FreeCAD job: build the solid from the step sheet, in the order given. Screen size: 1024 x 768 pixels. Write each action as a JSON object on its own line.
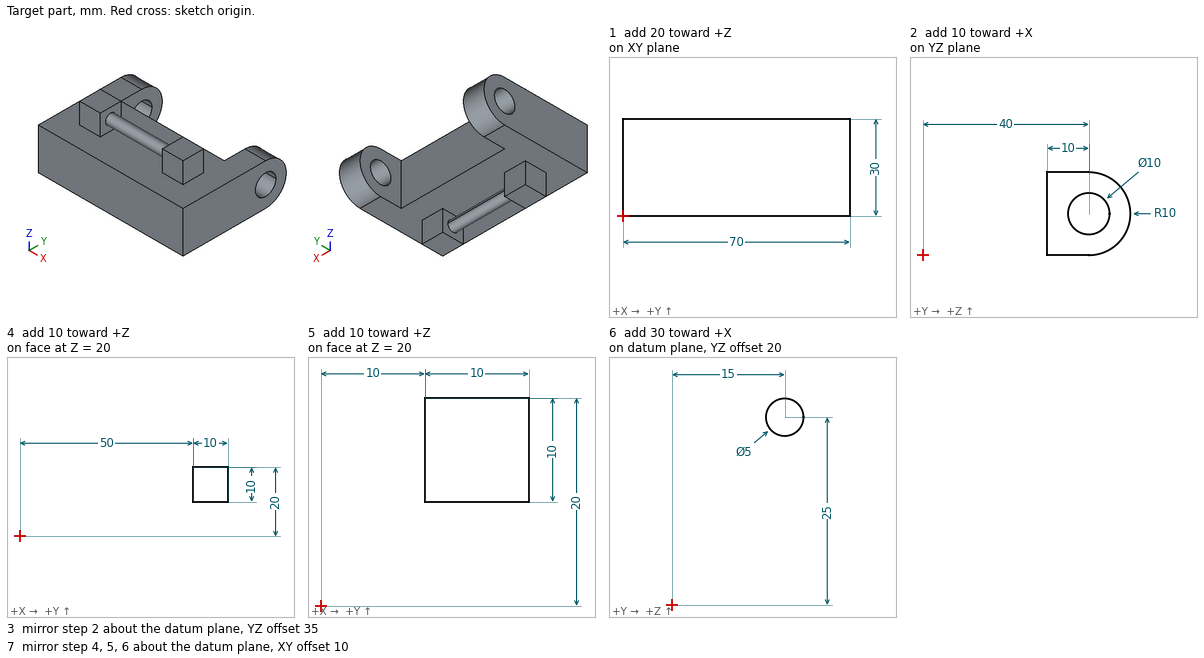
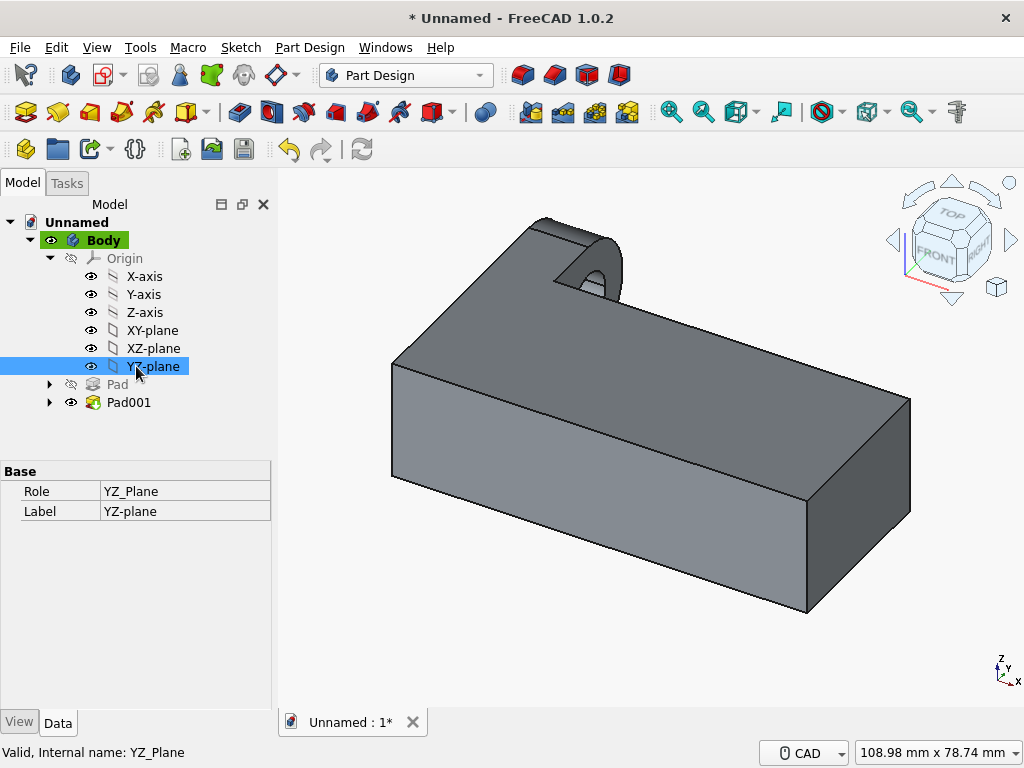
{"action": "left_click", "coordinate": [276, 76]}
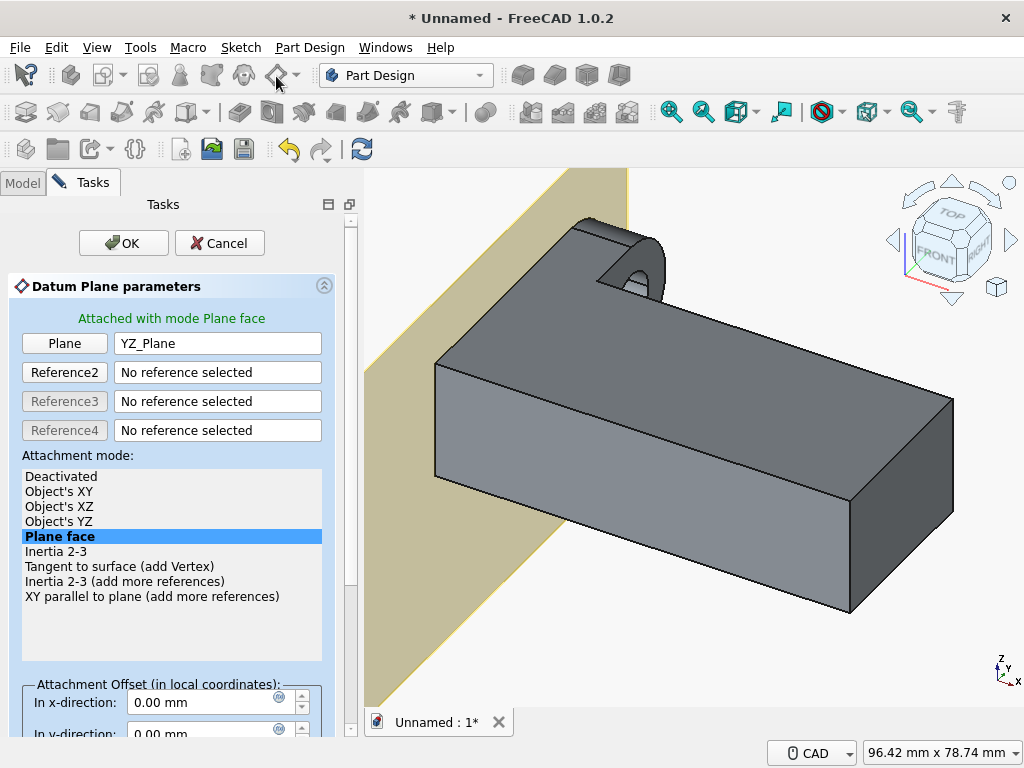
{"action": "scroll", "coordinate": [351, 475], "scroll_direction": "down", "scroll_amount": 2}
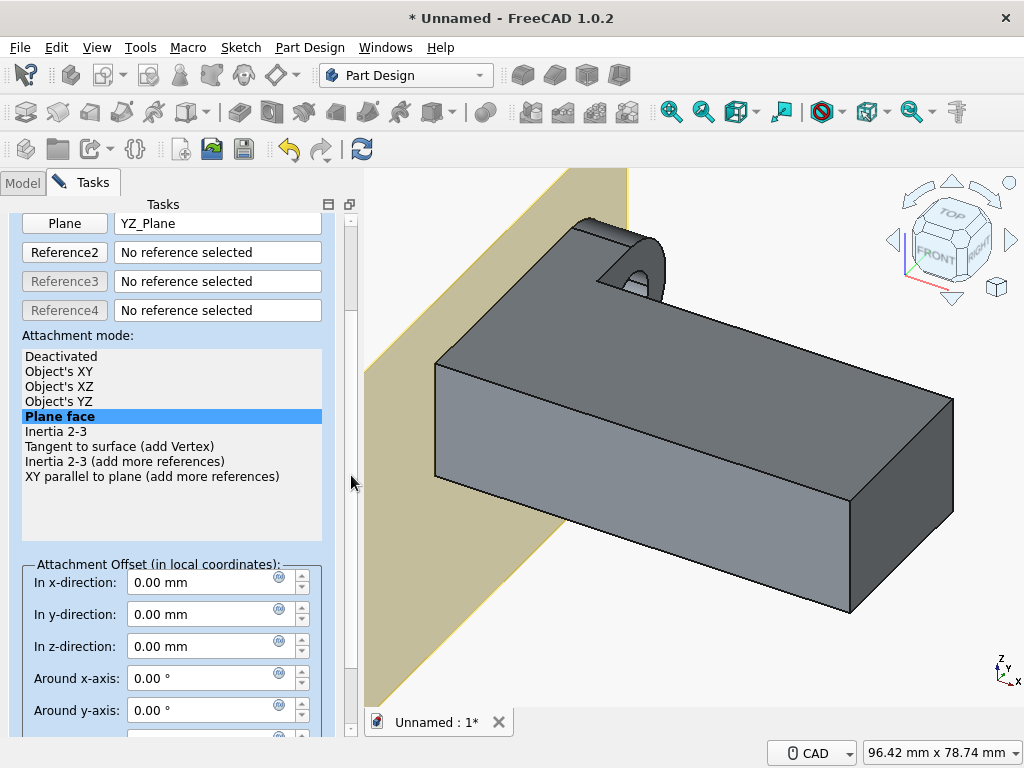
{"action": "triple_click", "coordinate": [210, 646]}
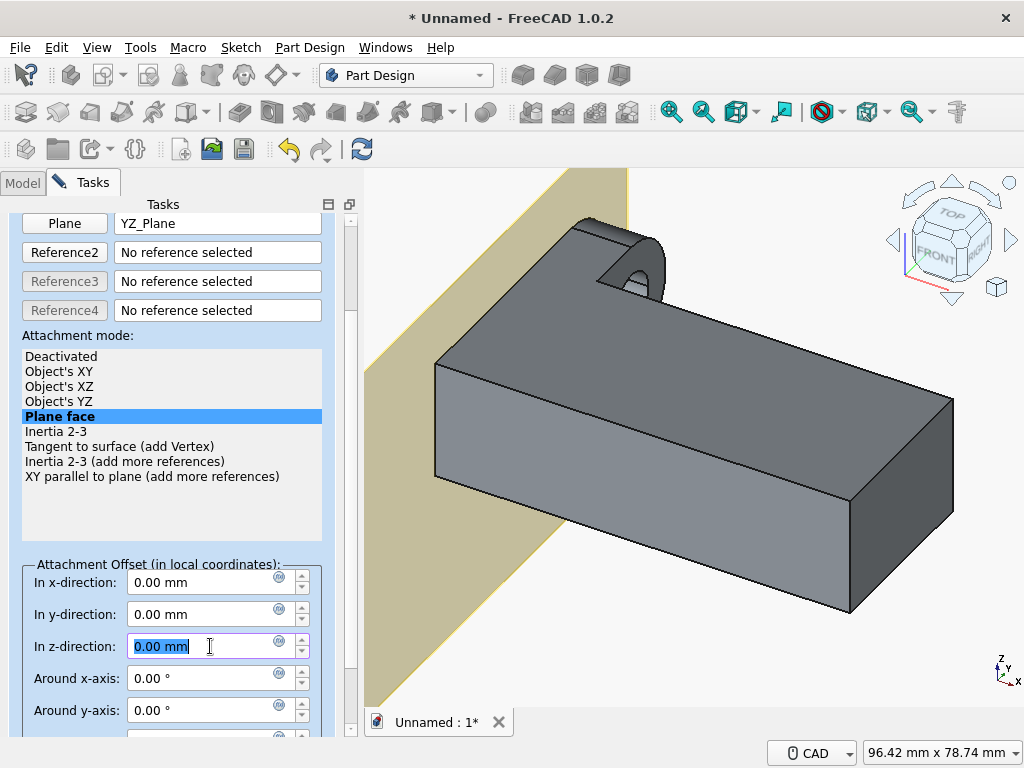
{"action": "type", "text": "35"}
{"action": "key", "text": "Tab"}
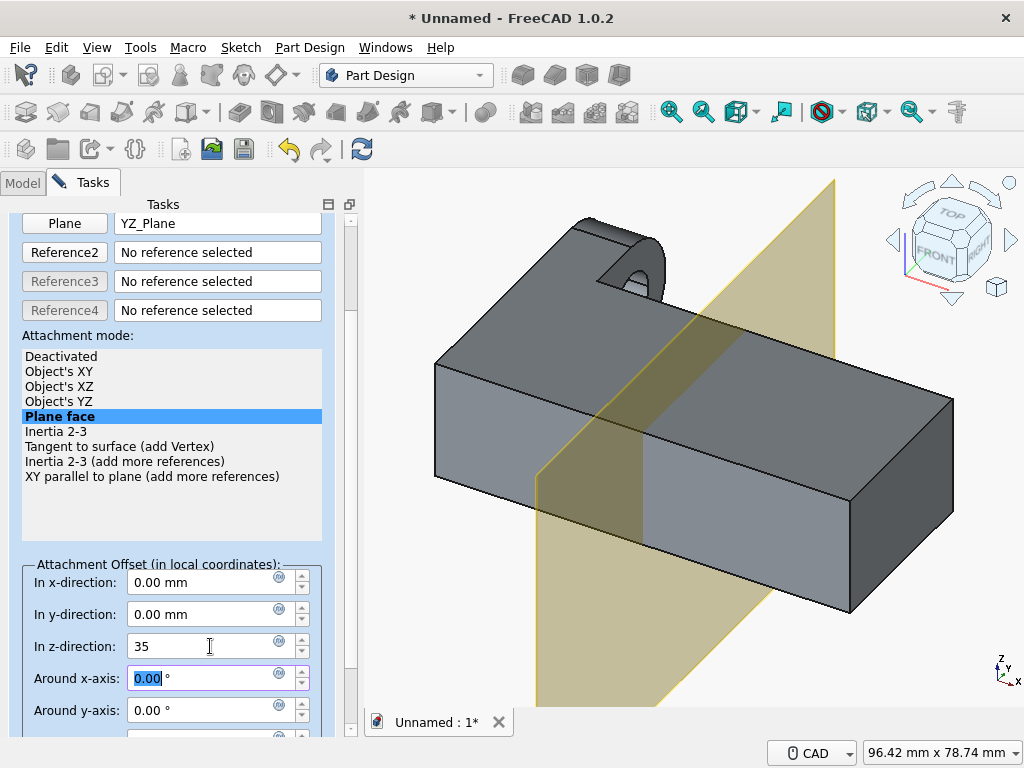
{"action": "scroll", "coordinate": [351, 475], "scroll_direction": "up", "scroll_amount": 3}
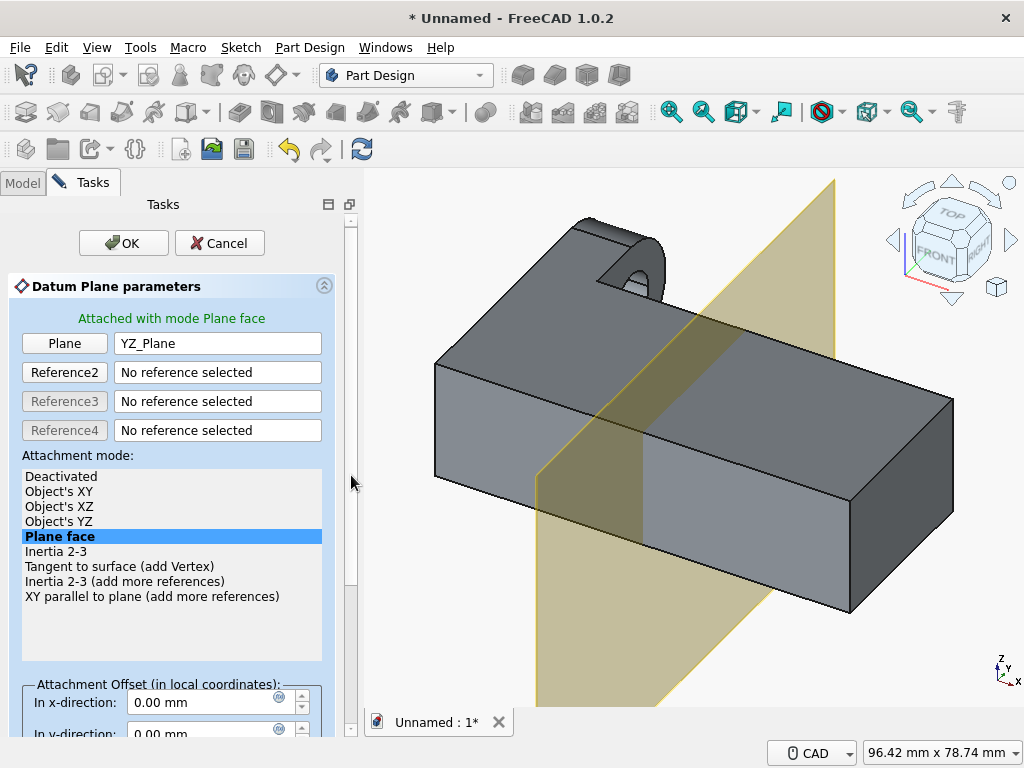
{"action": "left_click", "coordinate": [124, 243]}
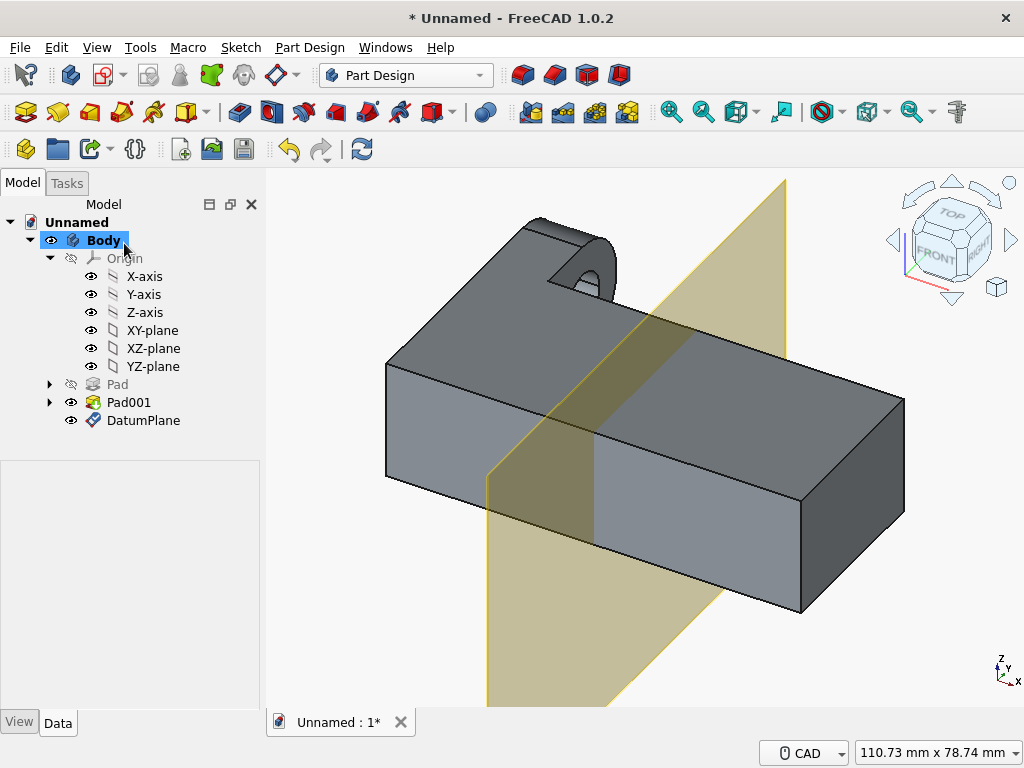
{"action": "left_click", "coordinate": [116, 402]}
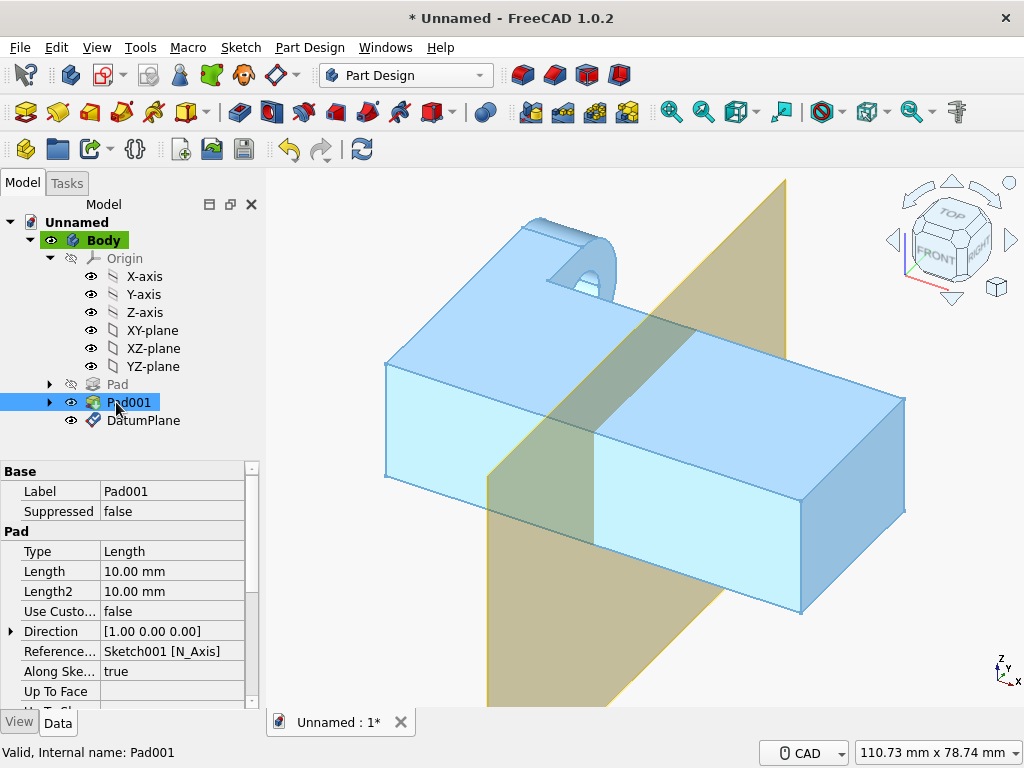
{"action": "left_click", "coordinate": [532, 112]}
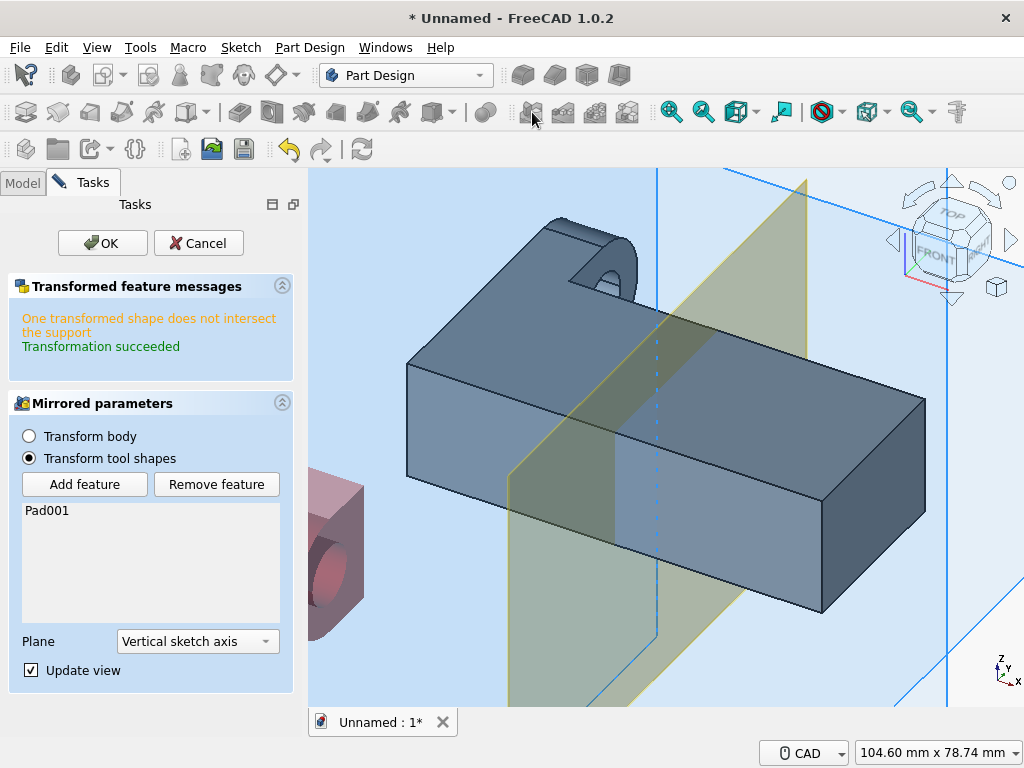
{"action": "left_click", "coordinate": [198, 642]}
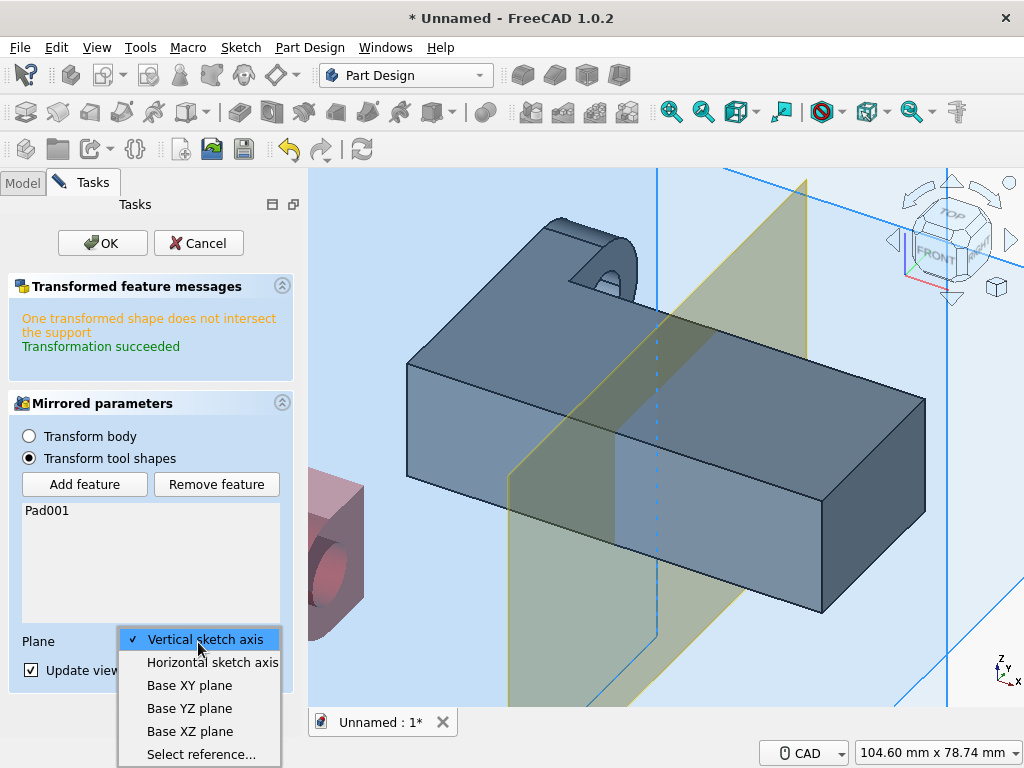
{"action": "left_click", "coordinate": [198, 754]}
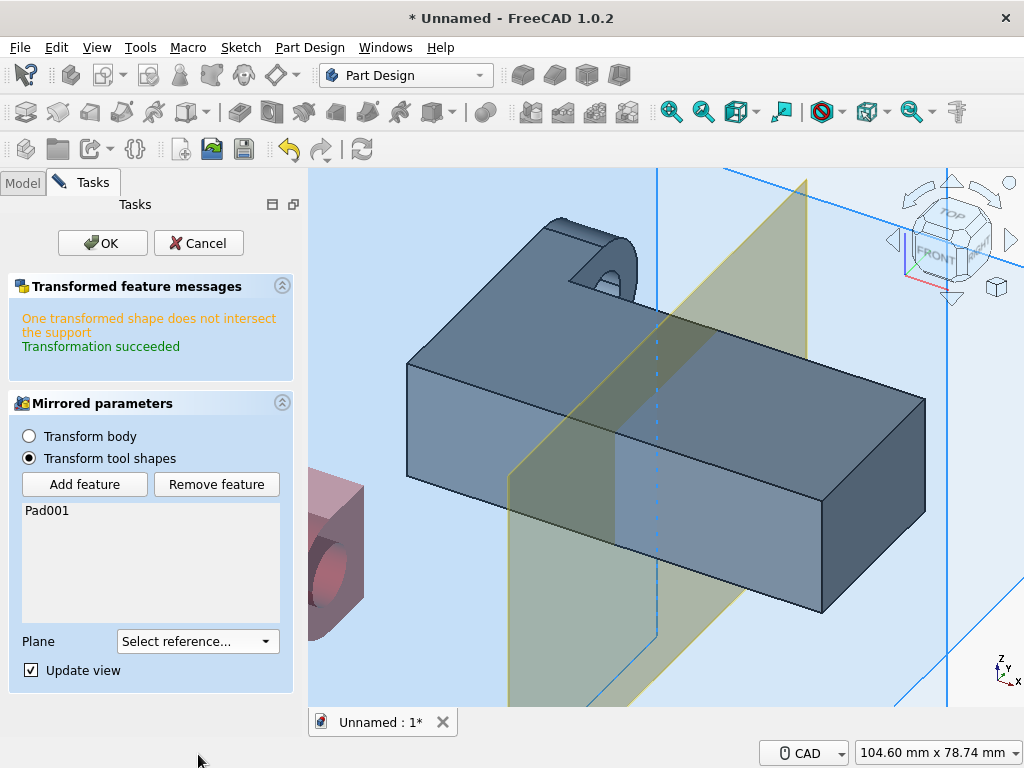
{"action": "left_click", "coordinate": [23, 182]}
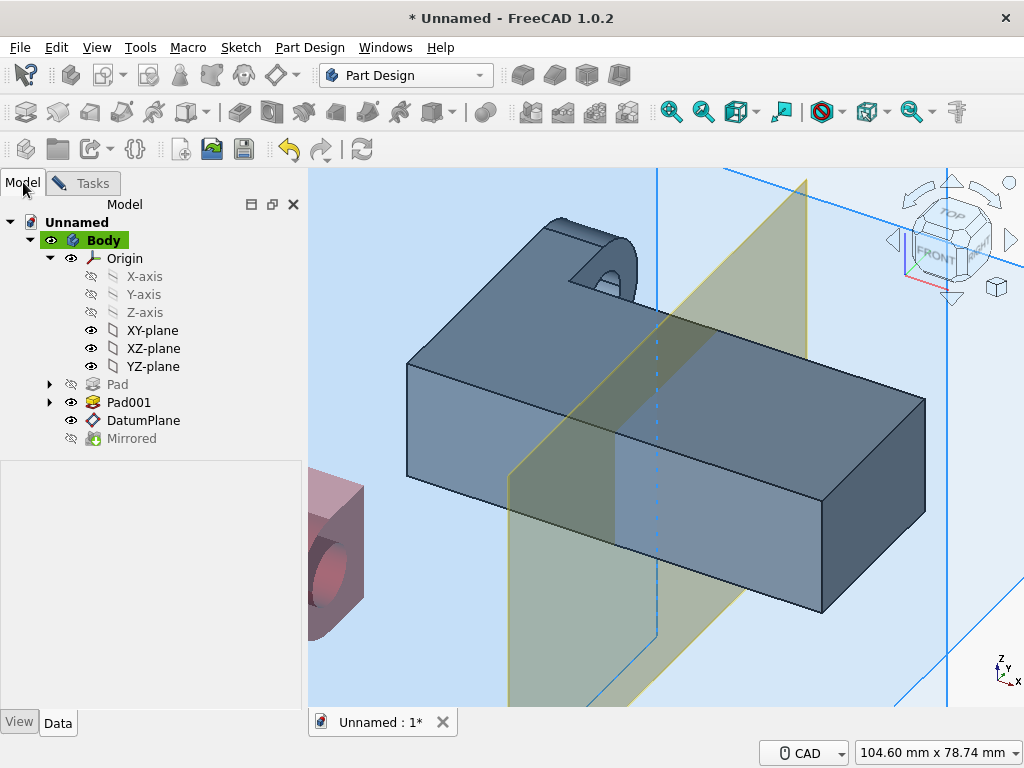
{"action": "left_click", "coordinate": [116, 420]}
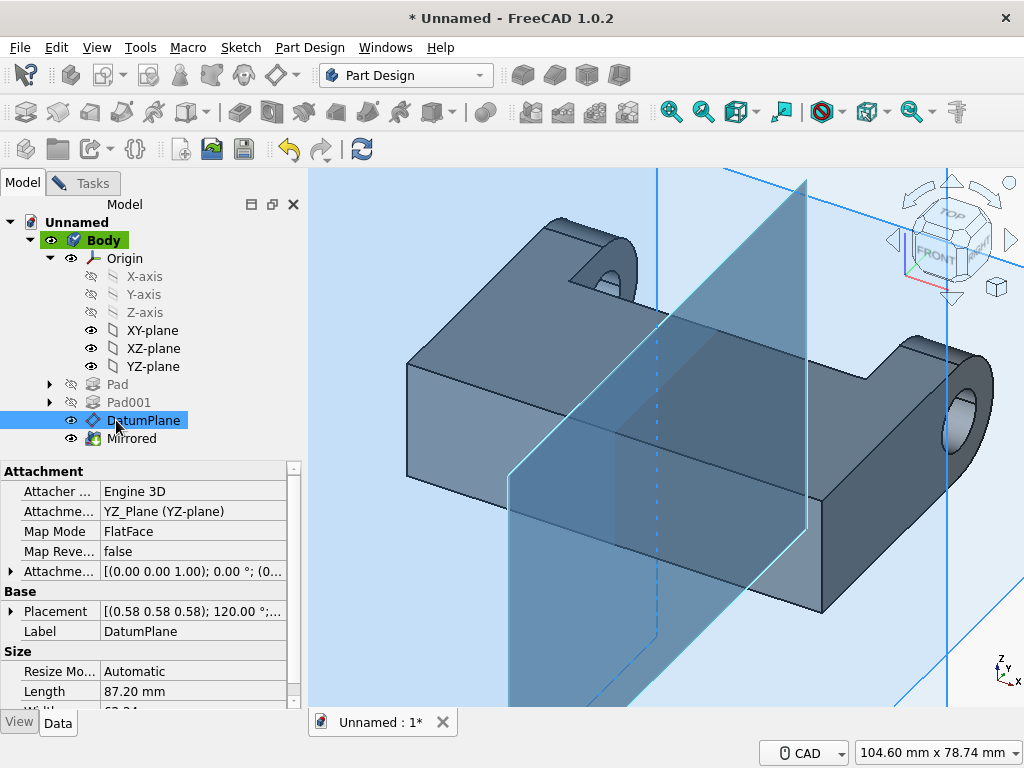
{"action": "left_click", "coordinate": [84, 182]}